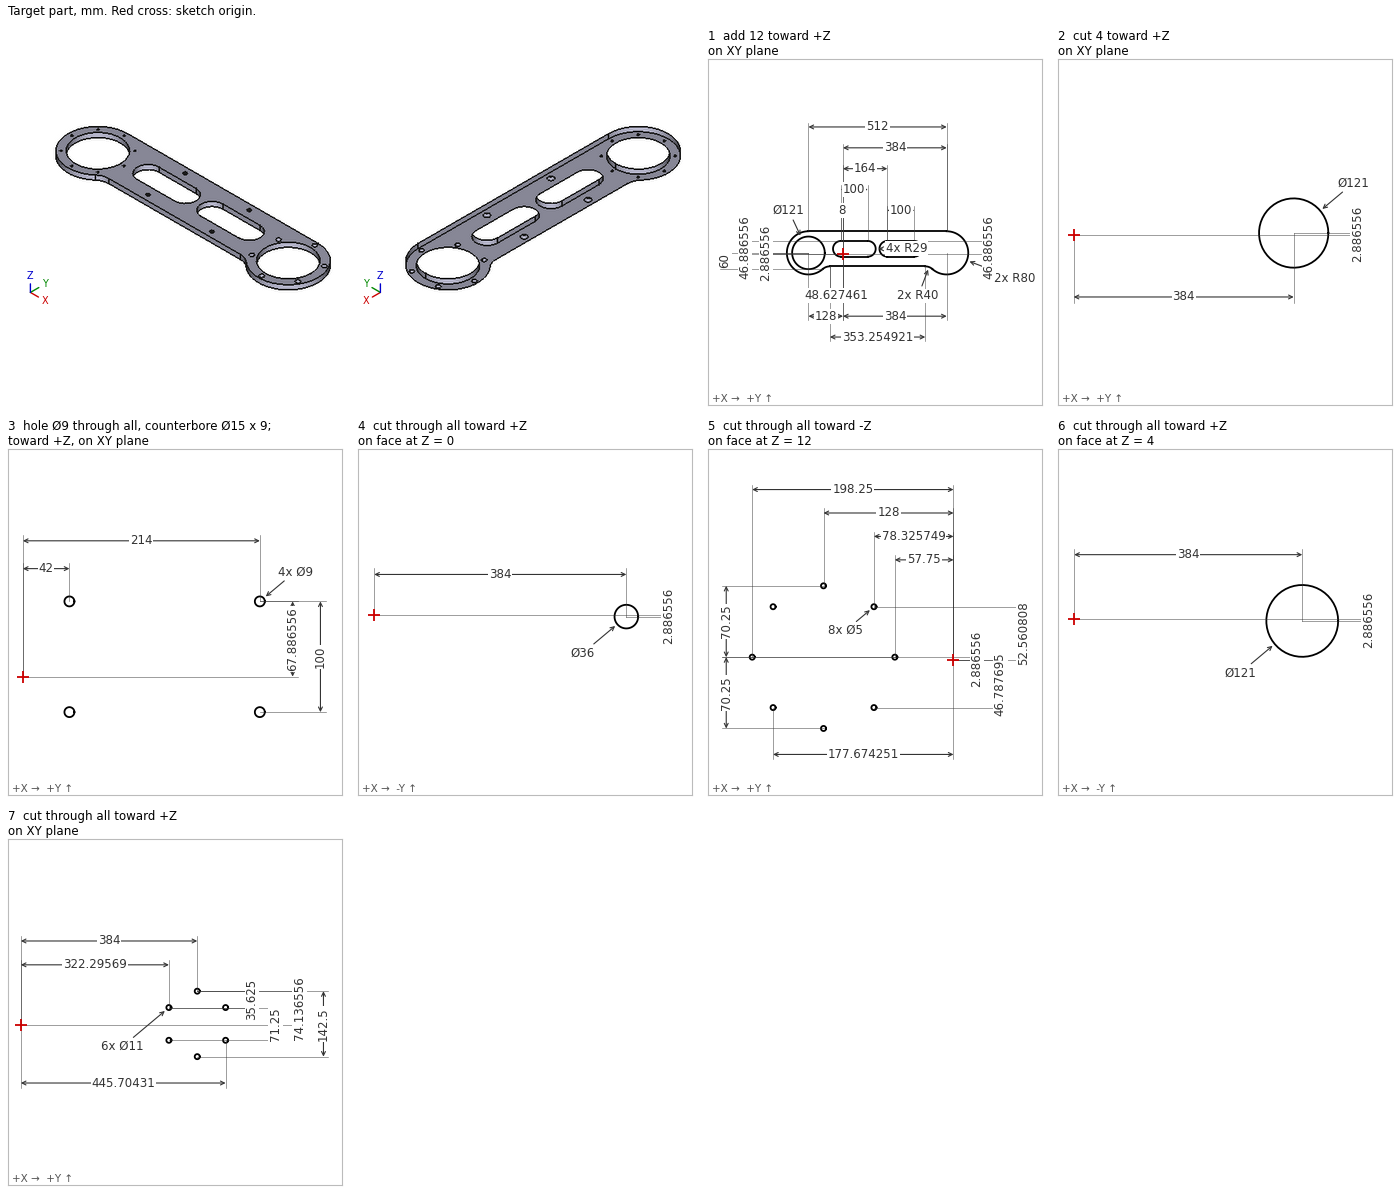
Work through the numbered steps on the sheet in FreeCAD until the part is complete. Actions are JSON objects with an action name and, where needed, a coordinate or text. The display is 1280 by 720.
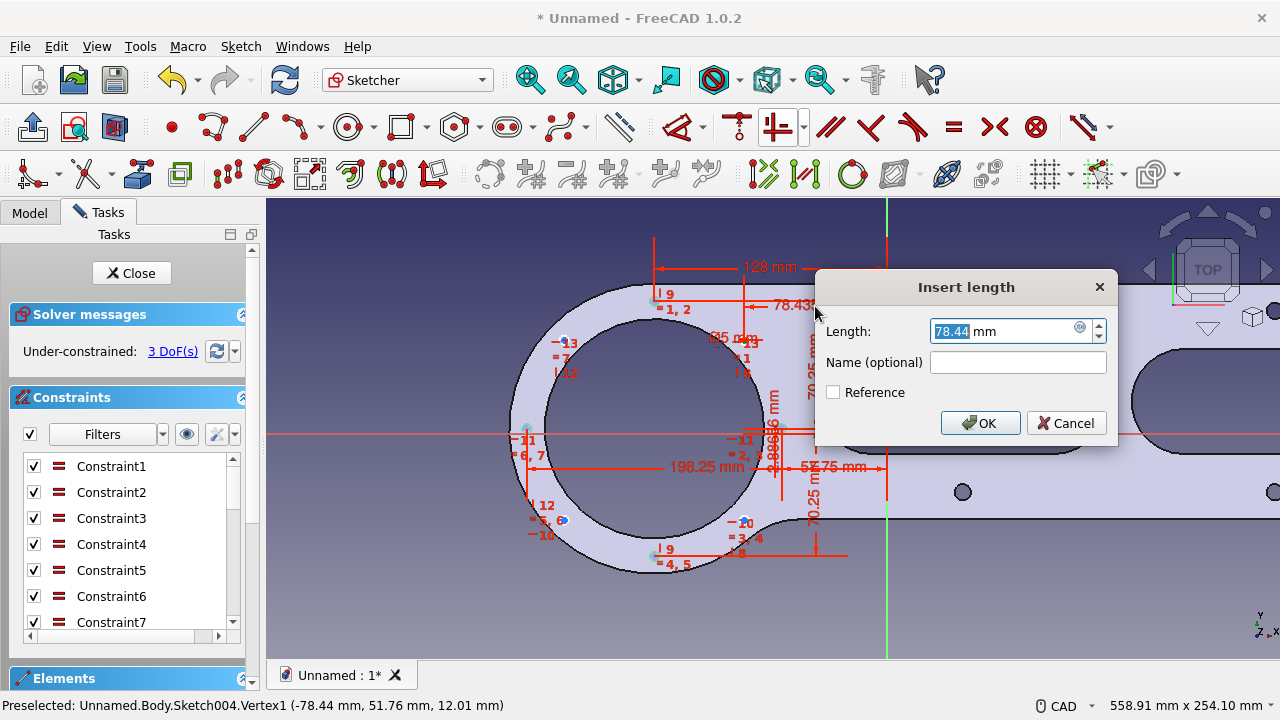
{"action": "type", "text": "78.325749"}
{"action": "key", "text": "Return"}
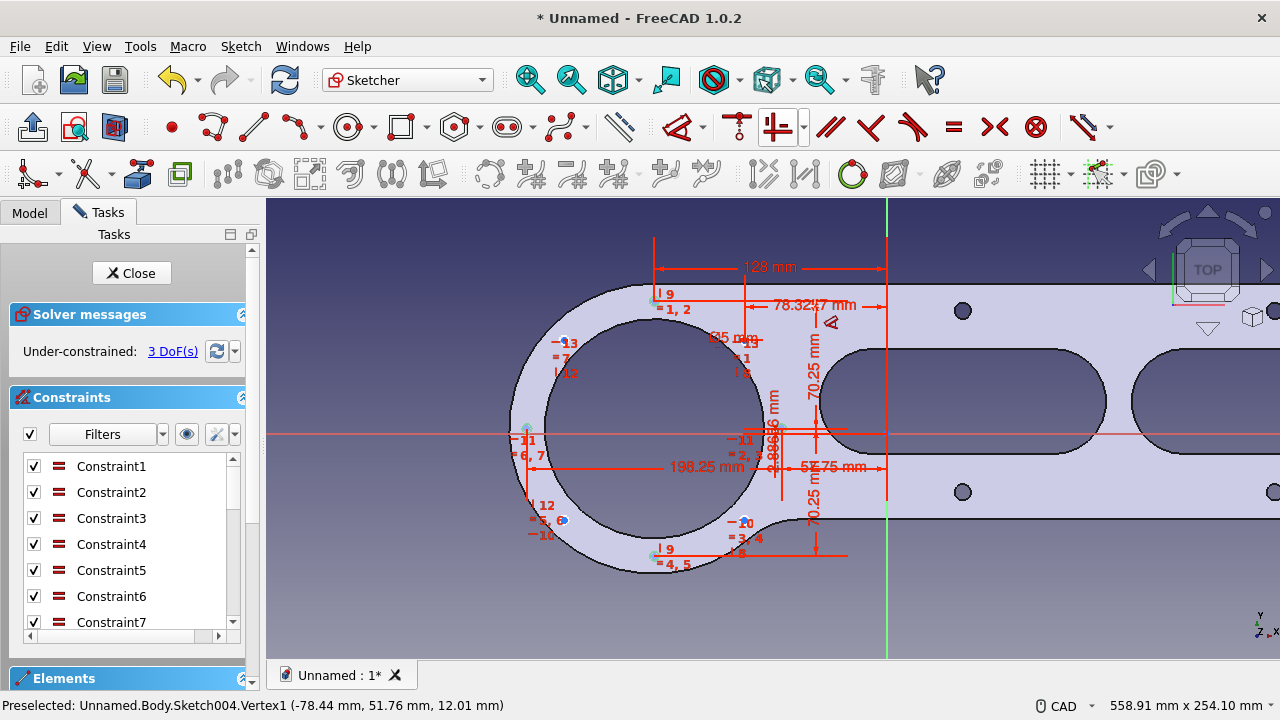
{"action": "left_click", "coordinate": [745, 340]}
{"action": "left_click", "coordinate": [921, 387]}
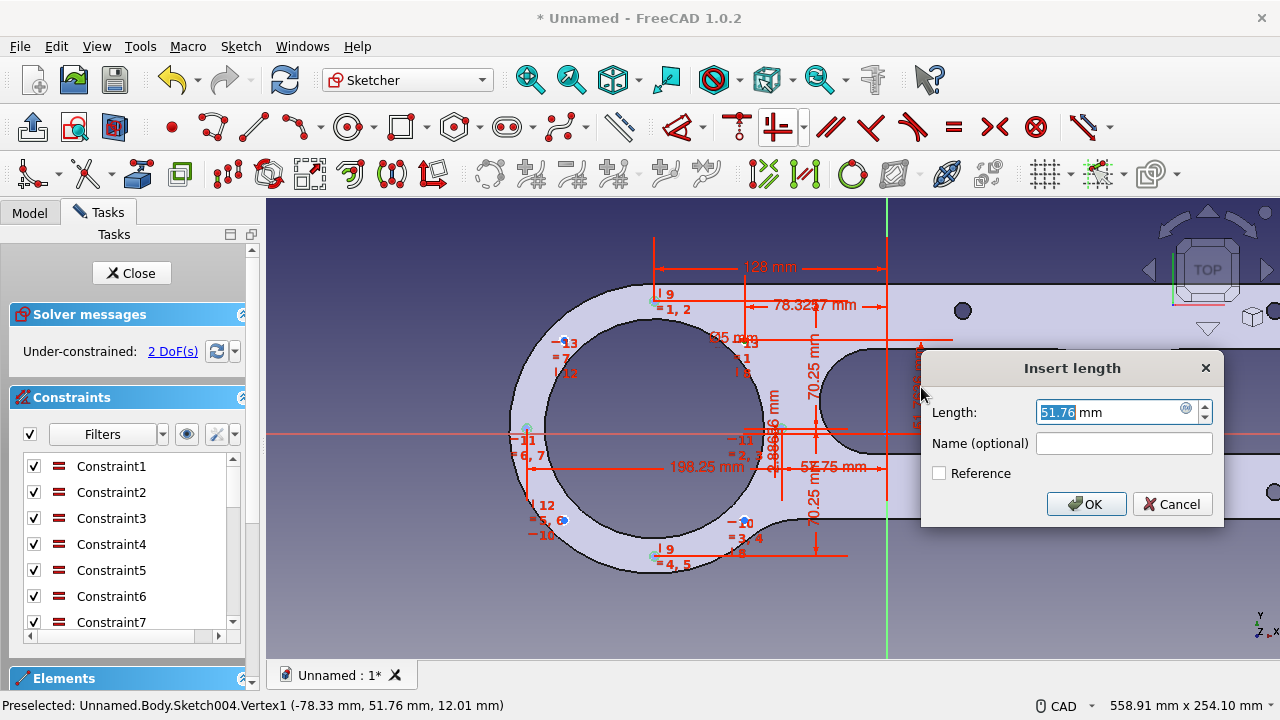
{"action": "type", "text": "52.560808"}
{"action": "key", "text": "Return"}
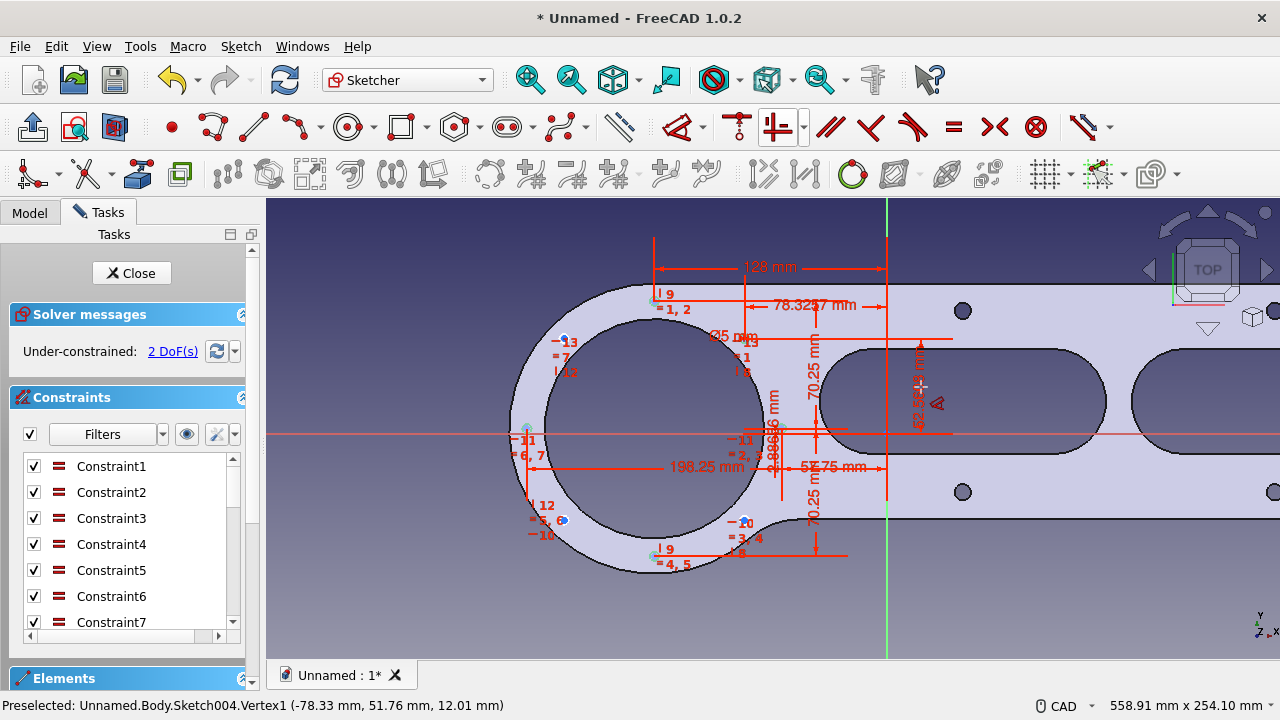
{"action": "left_click", "coordinate": [745, 520]}
{"action": "left_click", "coordinate": [921, 477]}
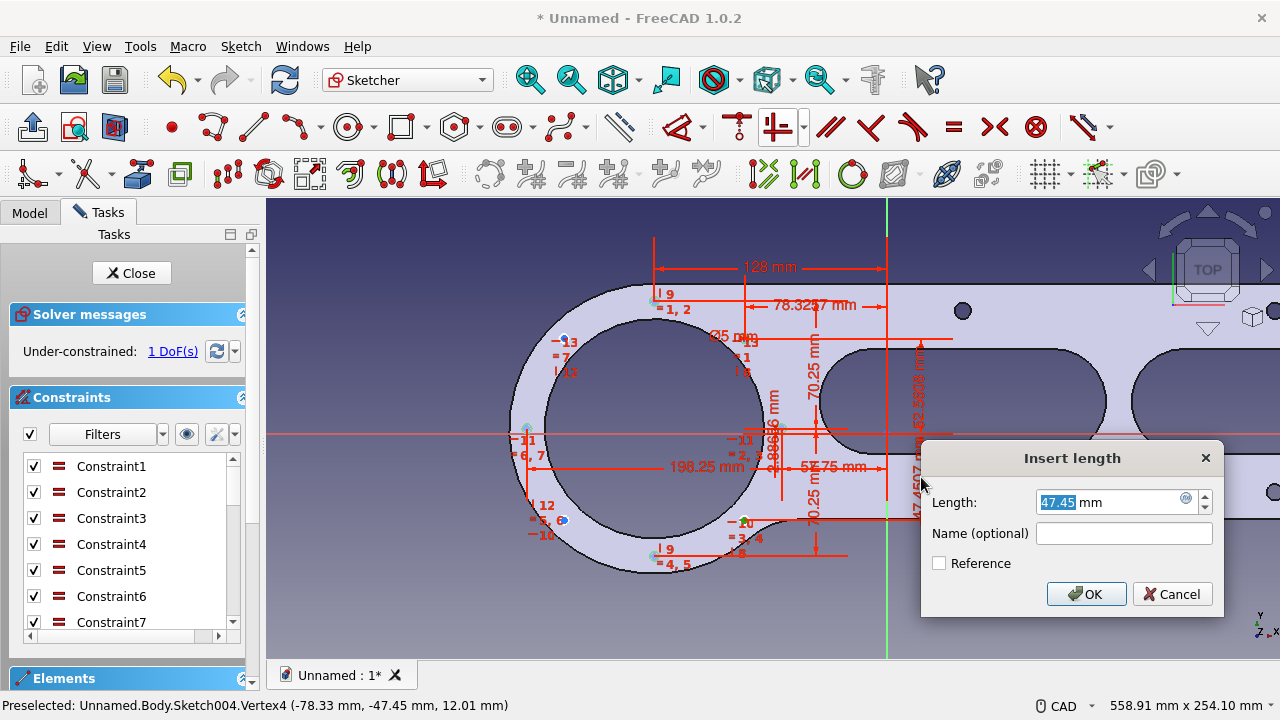
{"action": "type", "text": "46.787695"}
{"action": "key", "text": "Return"}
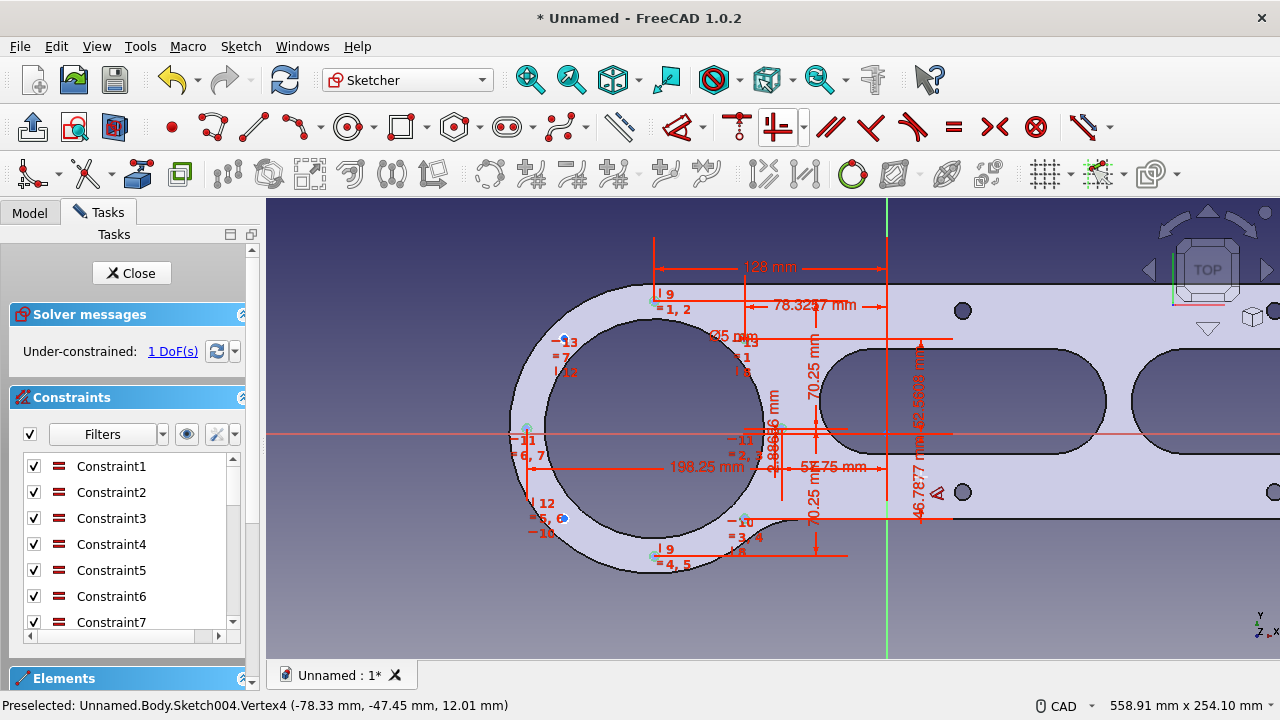
{"action": "left_click", "coordinate": [564, 519]}
{"action": "left_click", "coordinate": [725, 553]}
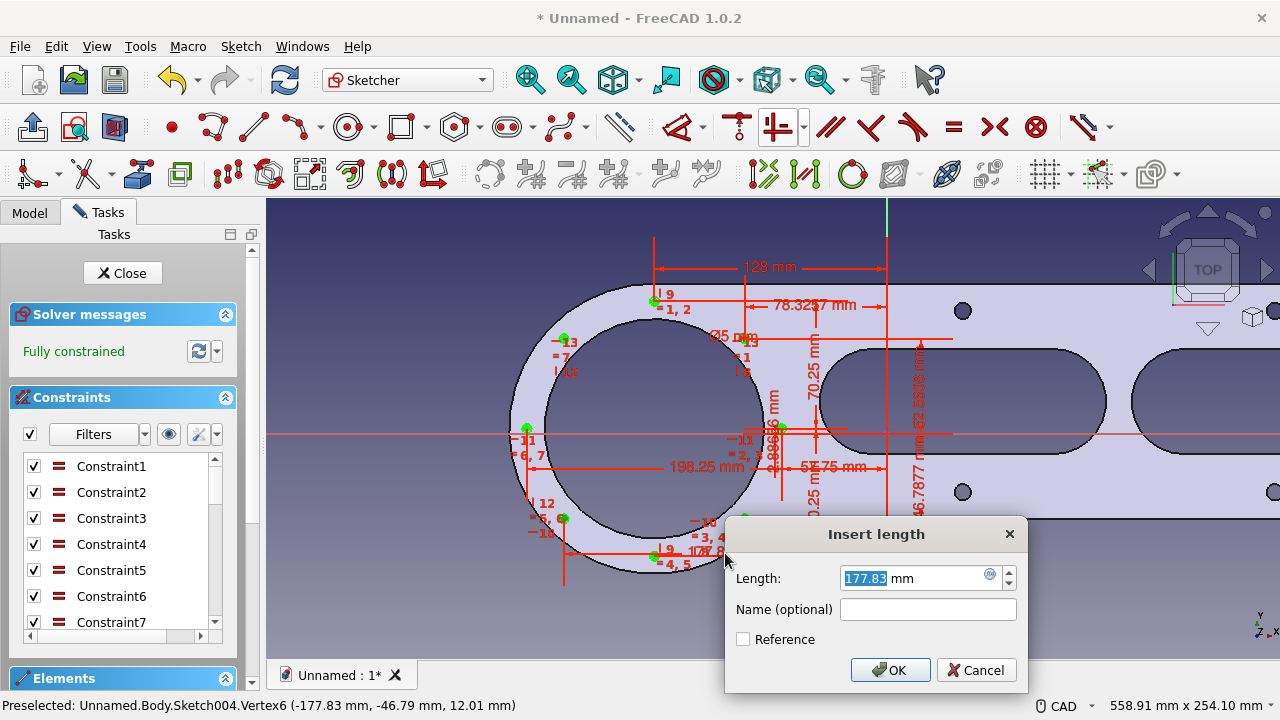
{"action": "type", "text": "177.674251"}
{"action": "key", "text": "Return"}
{"action": "key", "text": "Escape"}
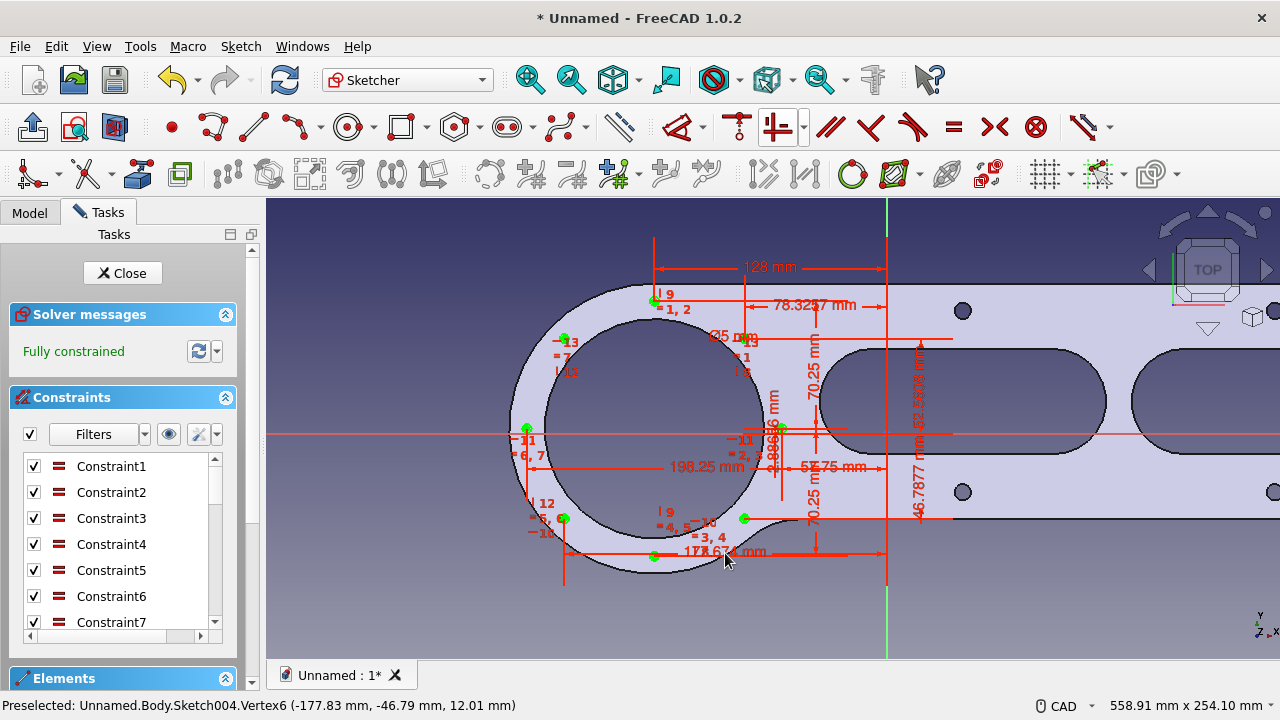
{"action": "left_click", "coordinate": [123, 273]}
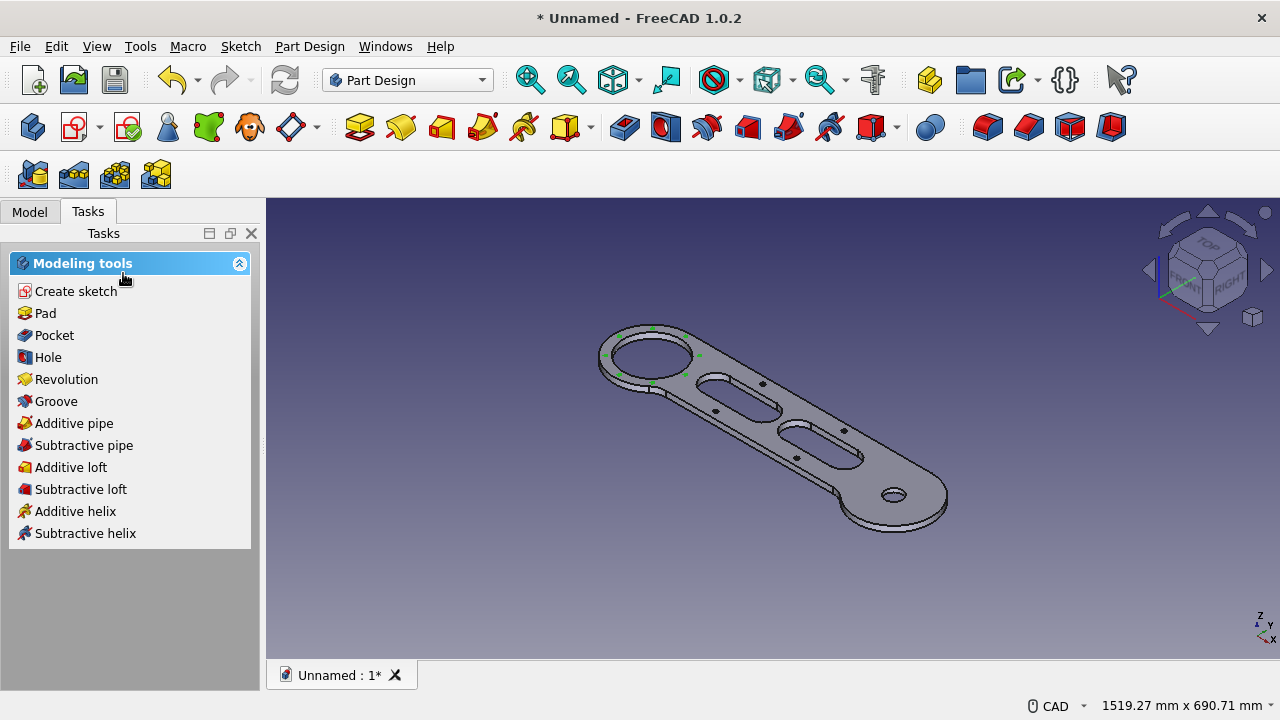
{"action": "left_click", "coordinate": [625, 128]}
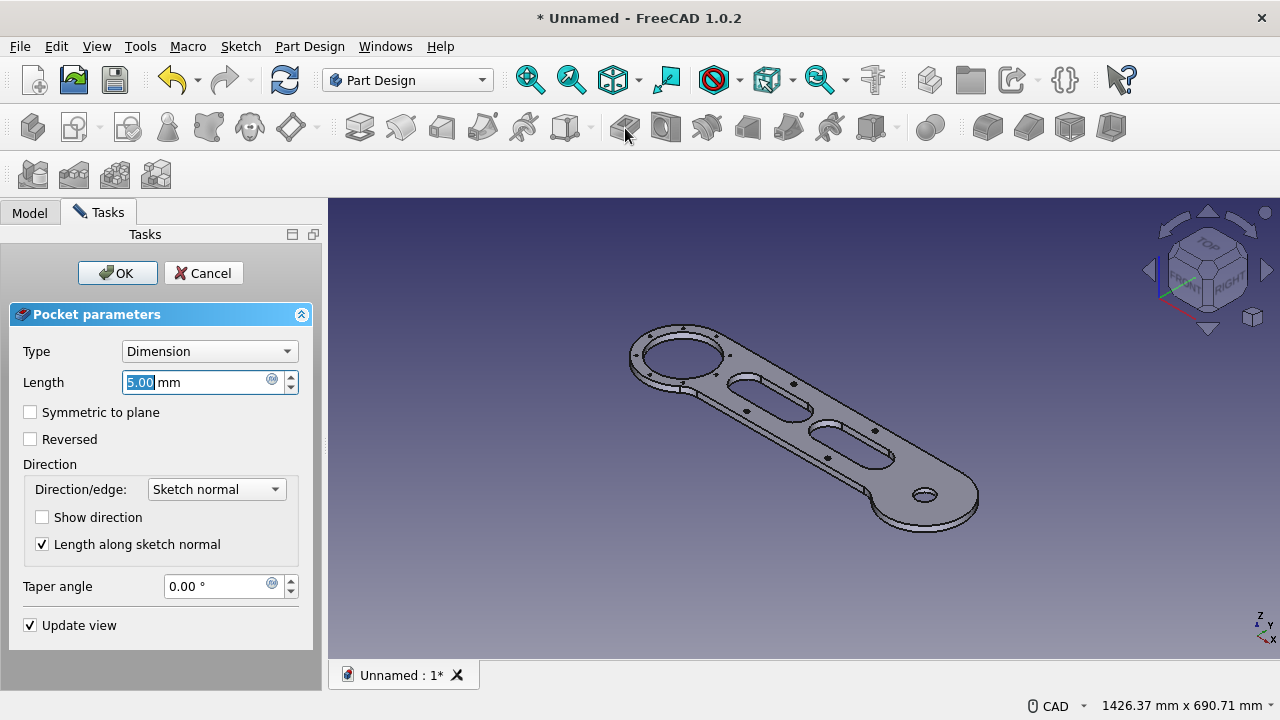
{"action": "left_click", "coordinate": [210, 352]}